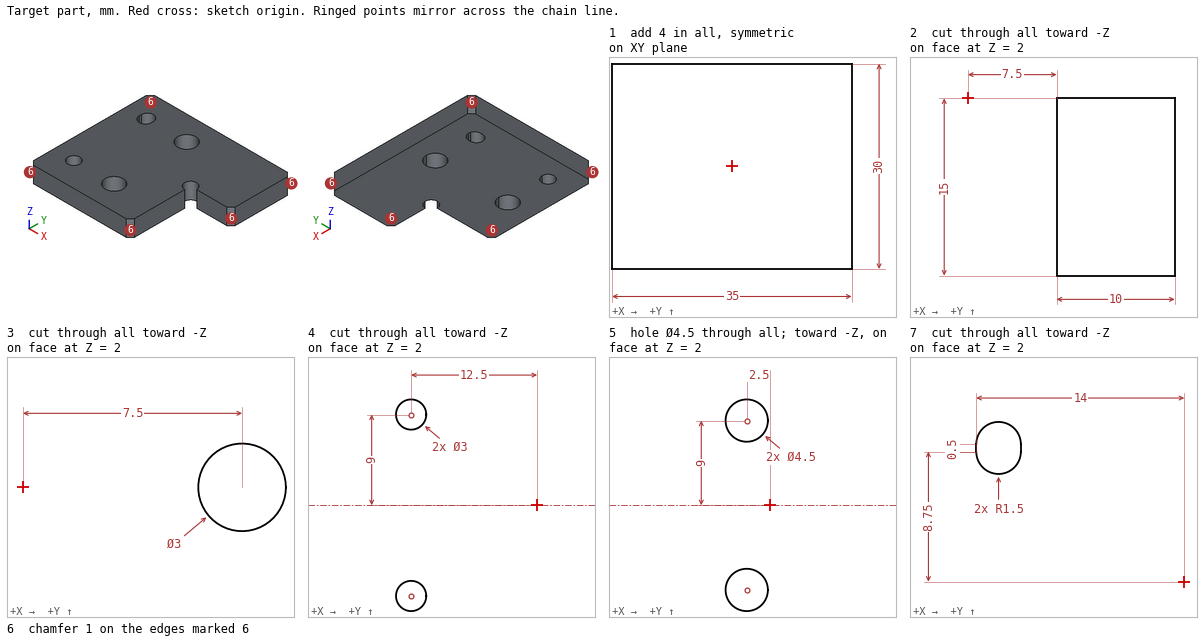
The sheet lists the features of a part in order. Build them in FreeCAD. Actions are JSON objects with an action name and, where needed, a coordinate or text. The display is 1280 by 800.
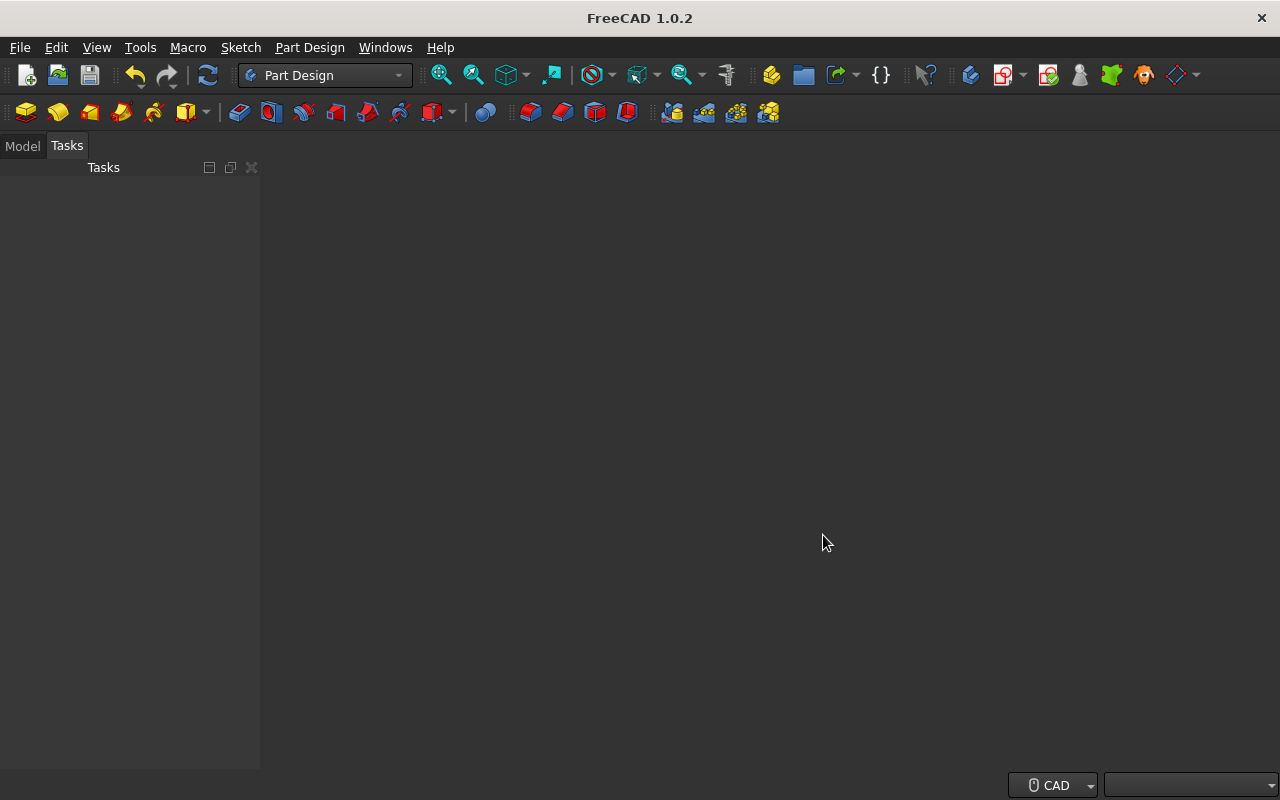
{"action": "key", "text": "ctrl+n"}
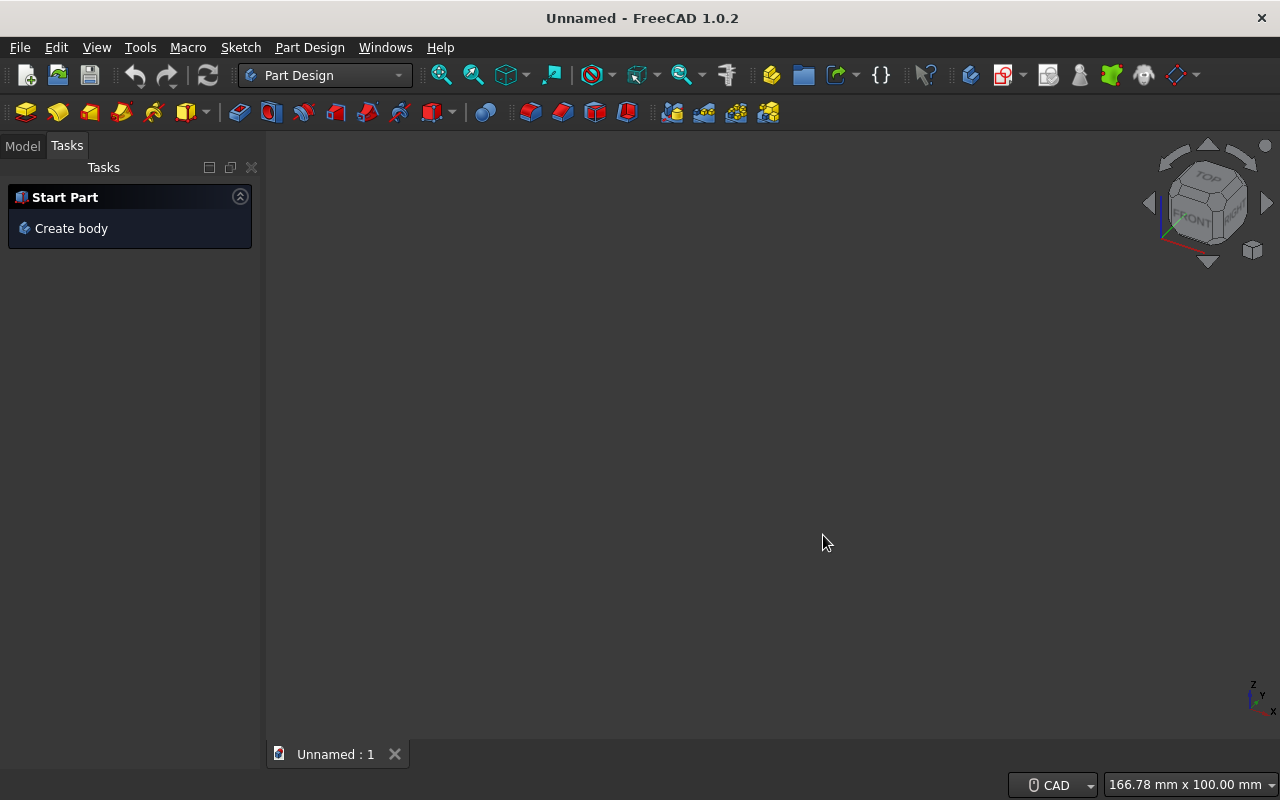
{"action": "left_click", "coordinate": [1004, 76]}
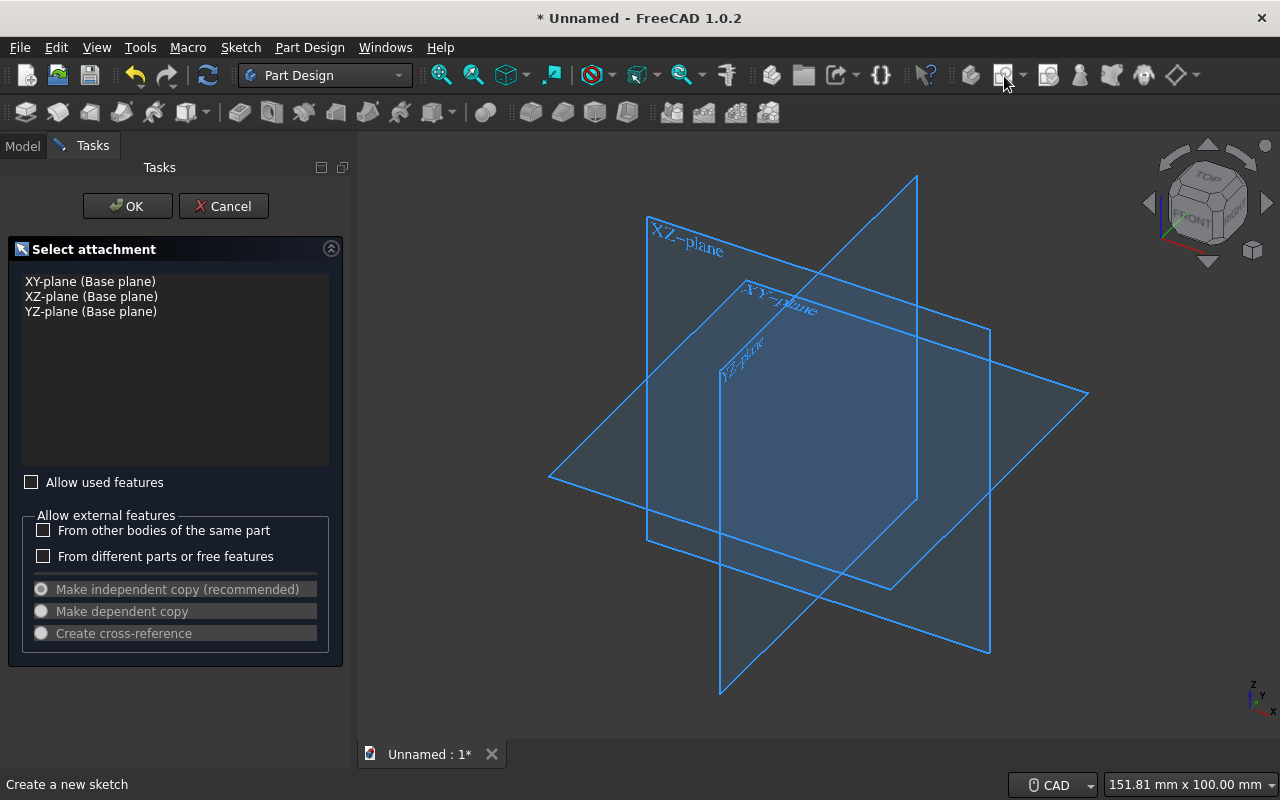
{"action": "left_click", "coordinate": [82, 282]}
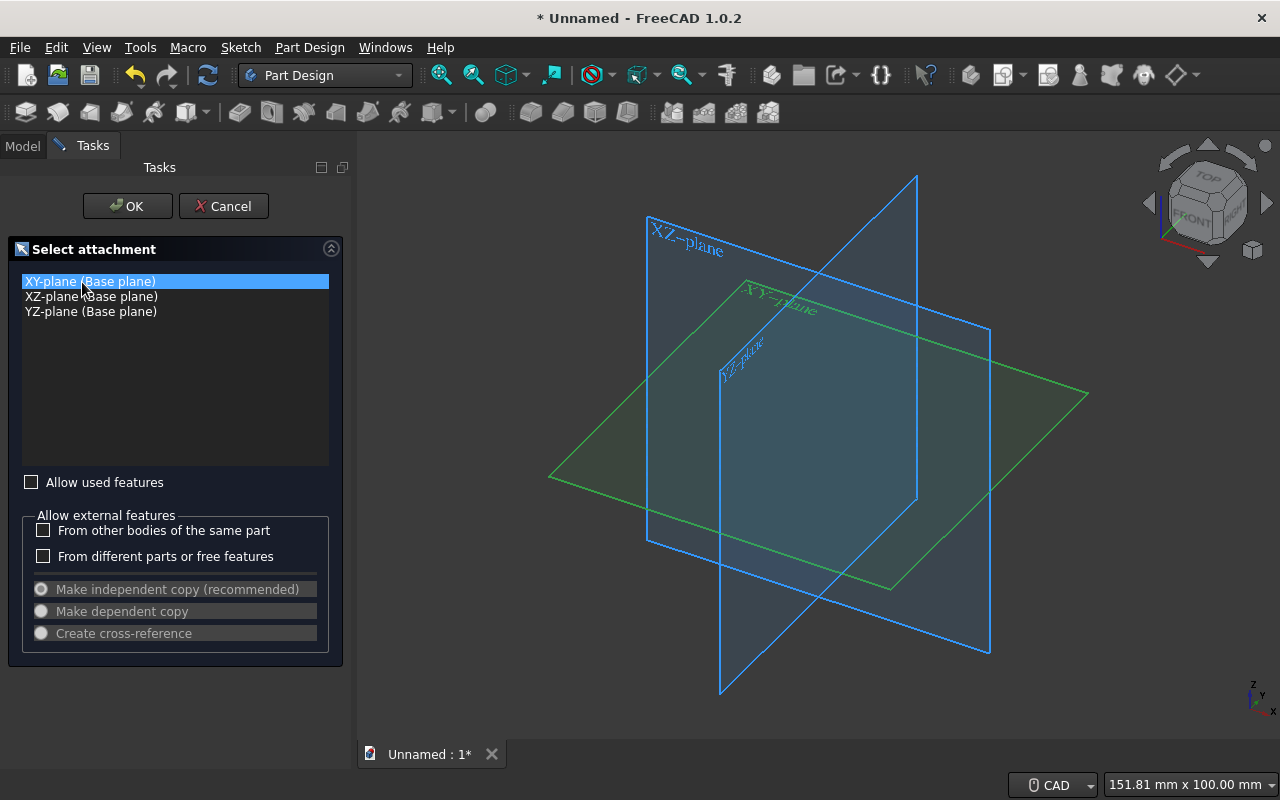
{"action": "left_click", "coordinate": [128, 206]}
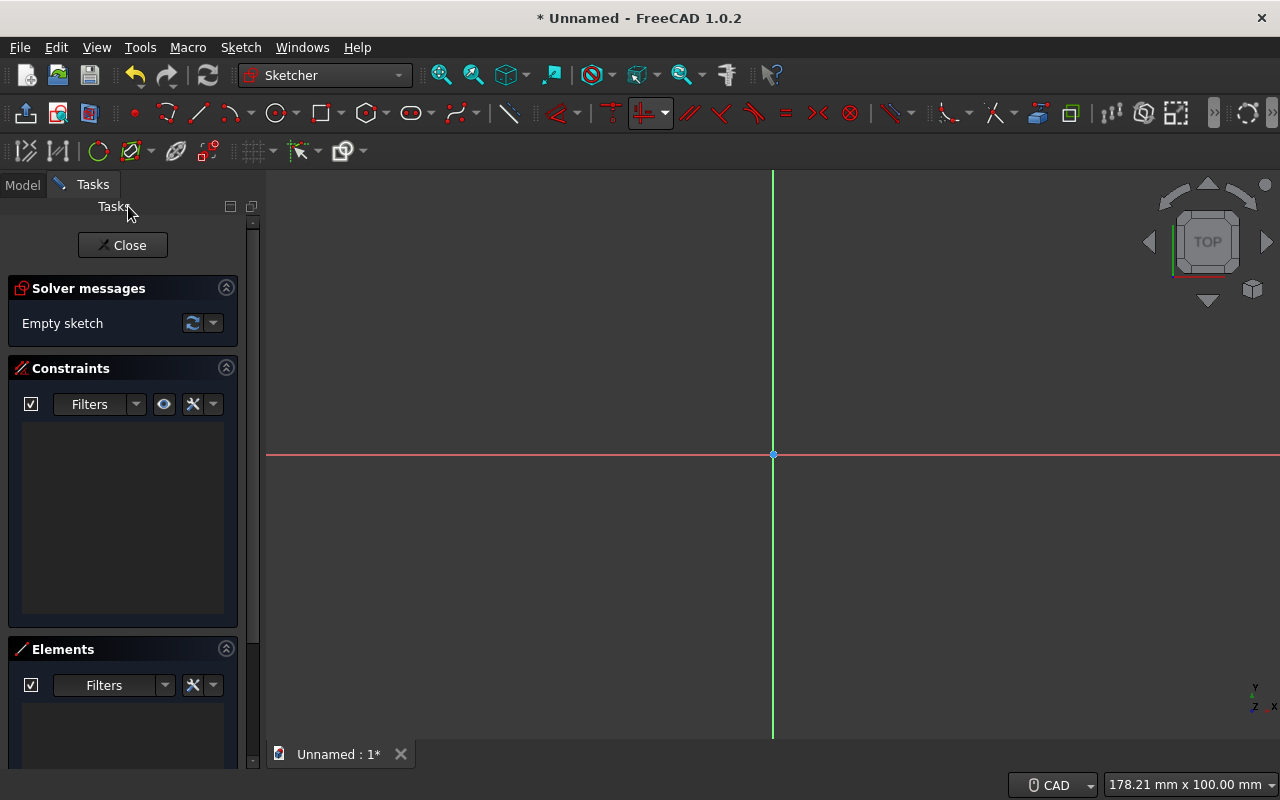
{"action": "scroll", "coordinate": [829, 455], "scroll_direction": "up", "scroll_amount": 4}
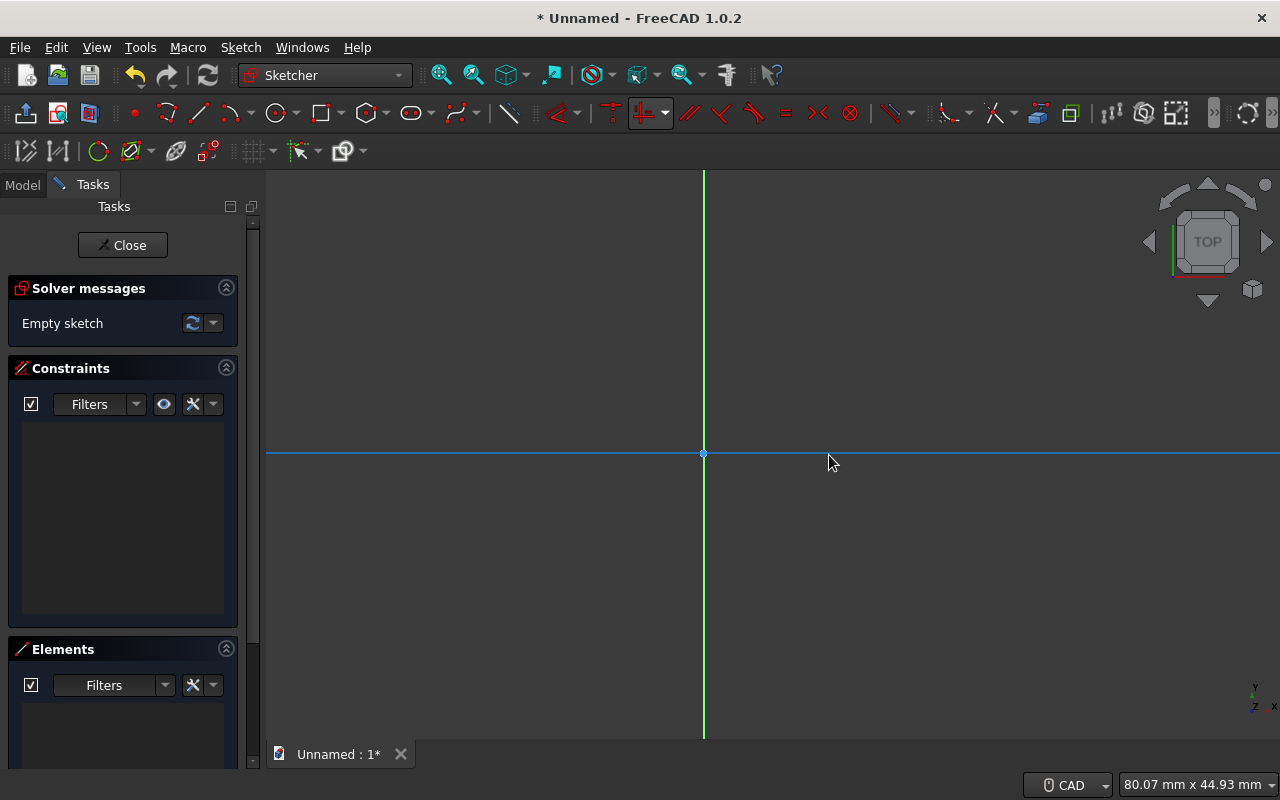
{"action": "key", "text": "g v"}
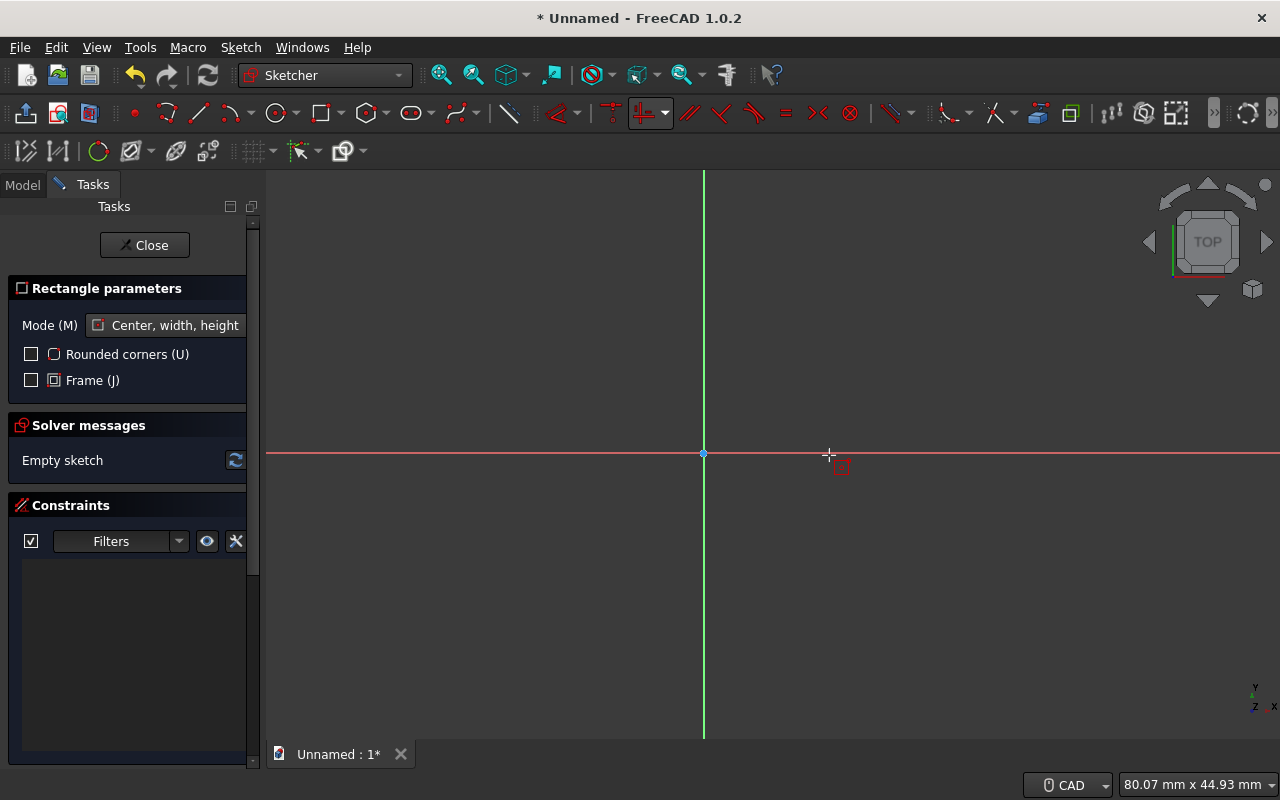
{"action": "left_click", "coordinate": [704, 453]}
{"action": "left_click", "coordinate": [925, 263]}
{"action": "key", "text": "Escape"}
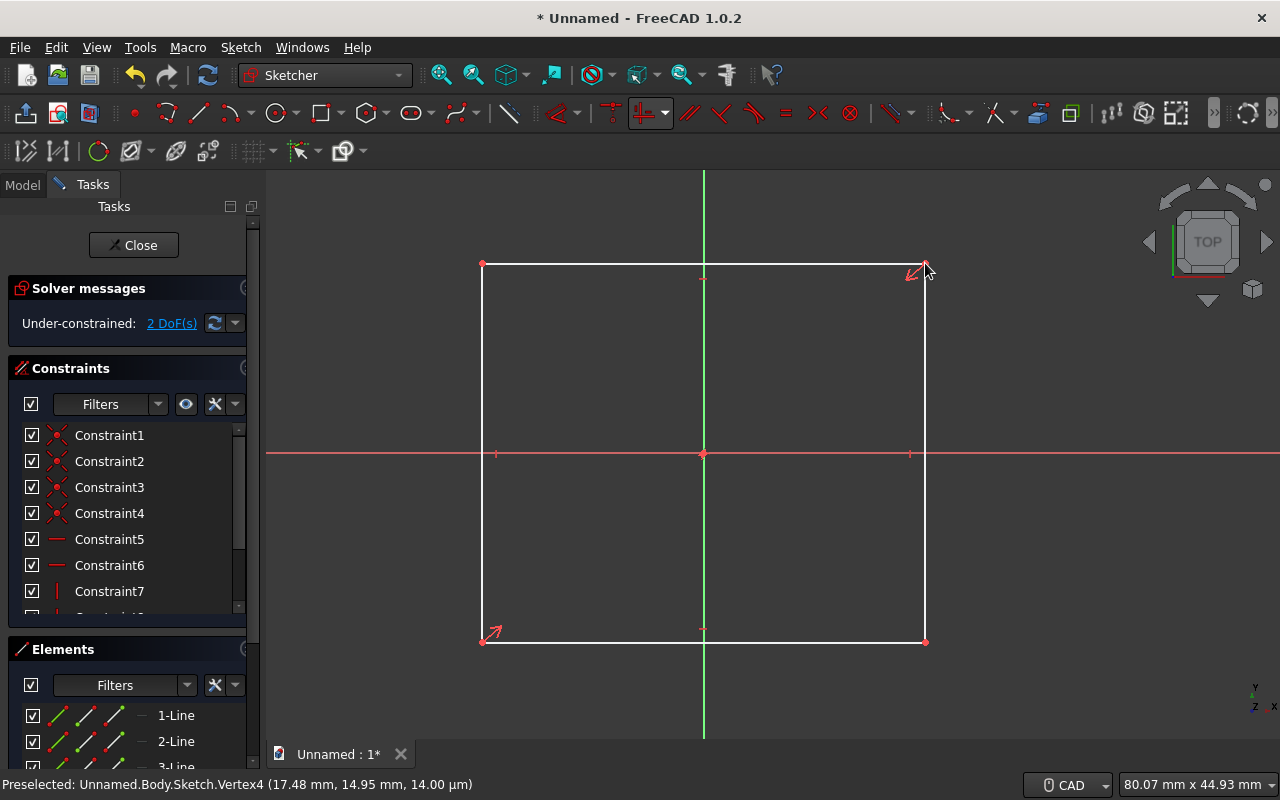
{"action": "left_click", "coordinate": [556, 114]}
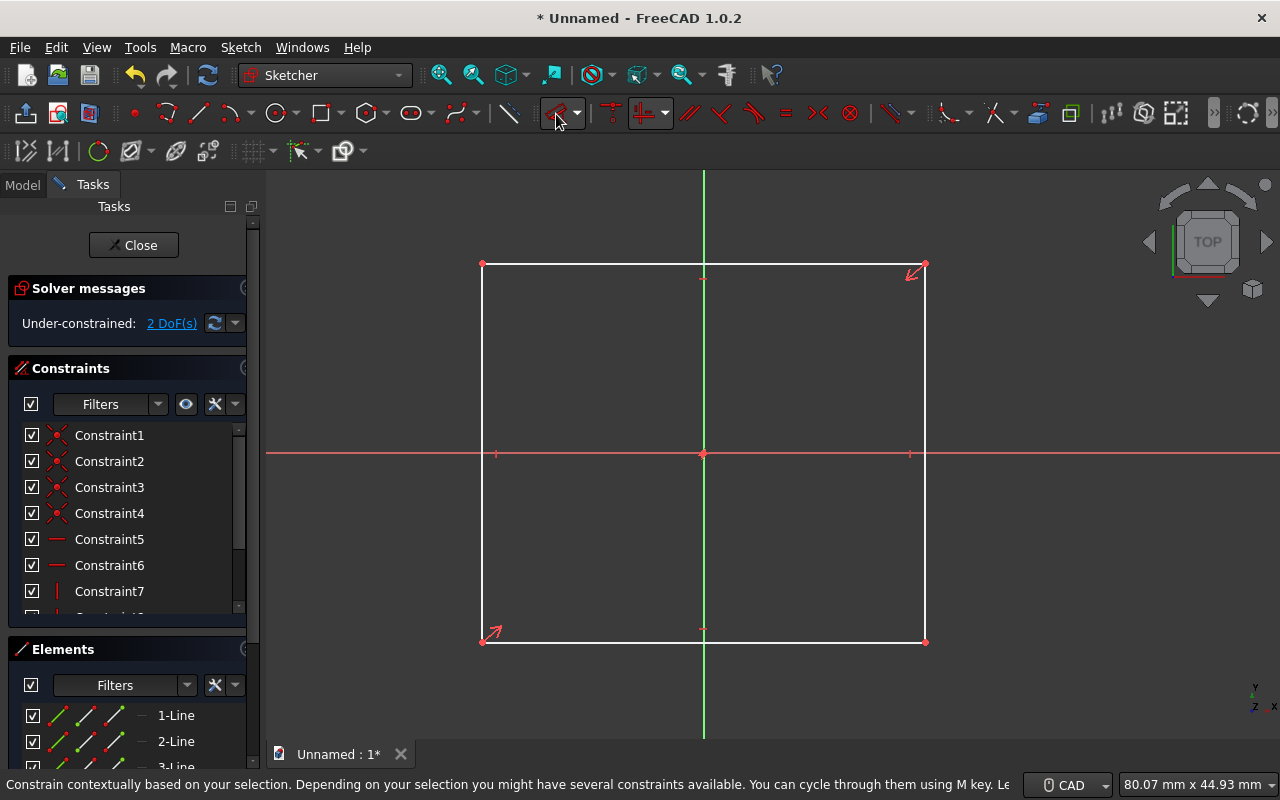
{"action": "left_click", "coordinate": [615, 643]}
{"action": "left_click", "coordinate": [602, 677]}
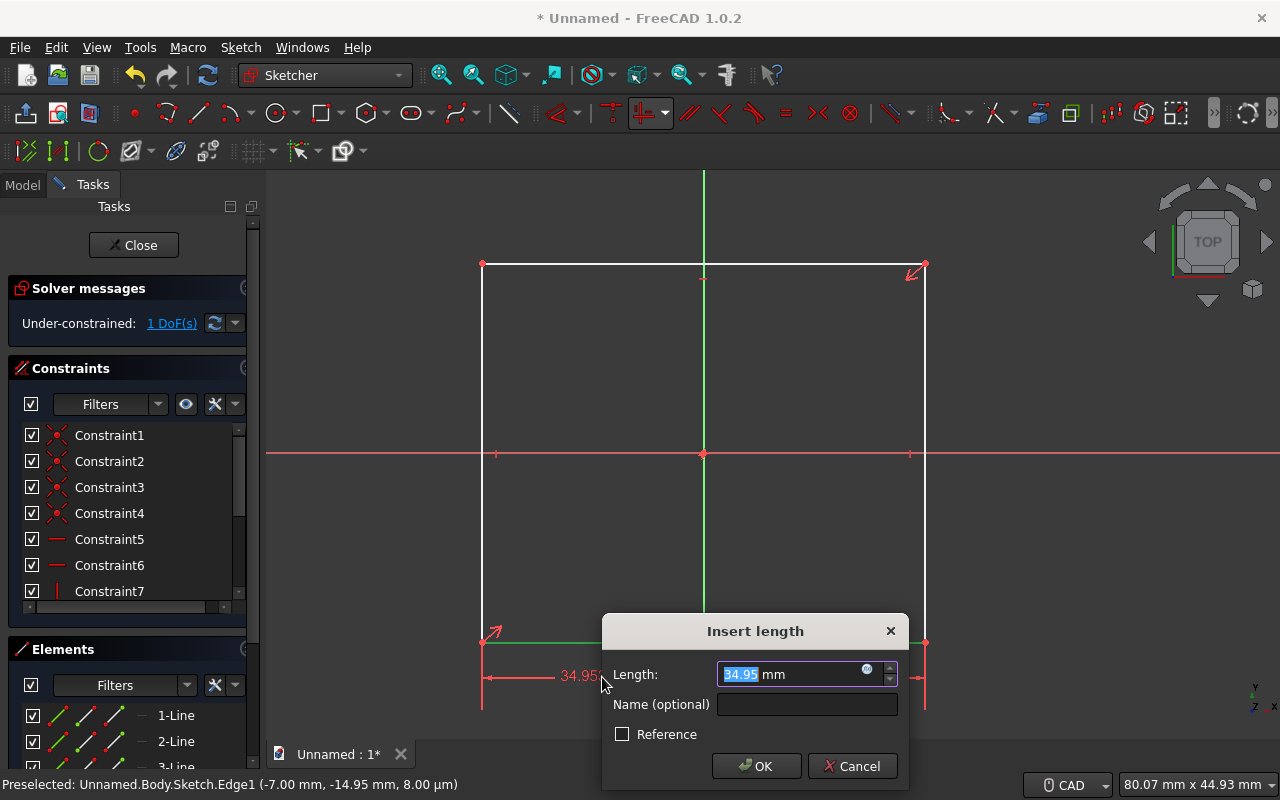
{"action": "type", "text": "35"}
{"action": "key", "text": "Return"}